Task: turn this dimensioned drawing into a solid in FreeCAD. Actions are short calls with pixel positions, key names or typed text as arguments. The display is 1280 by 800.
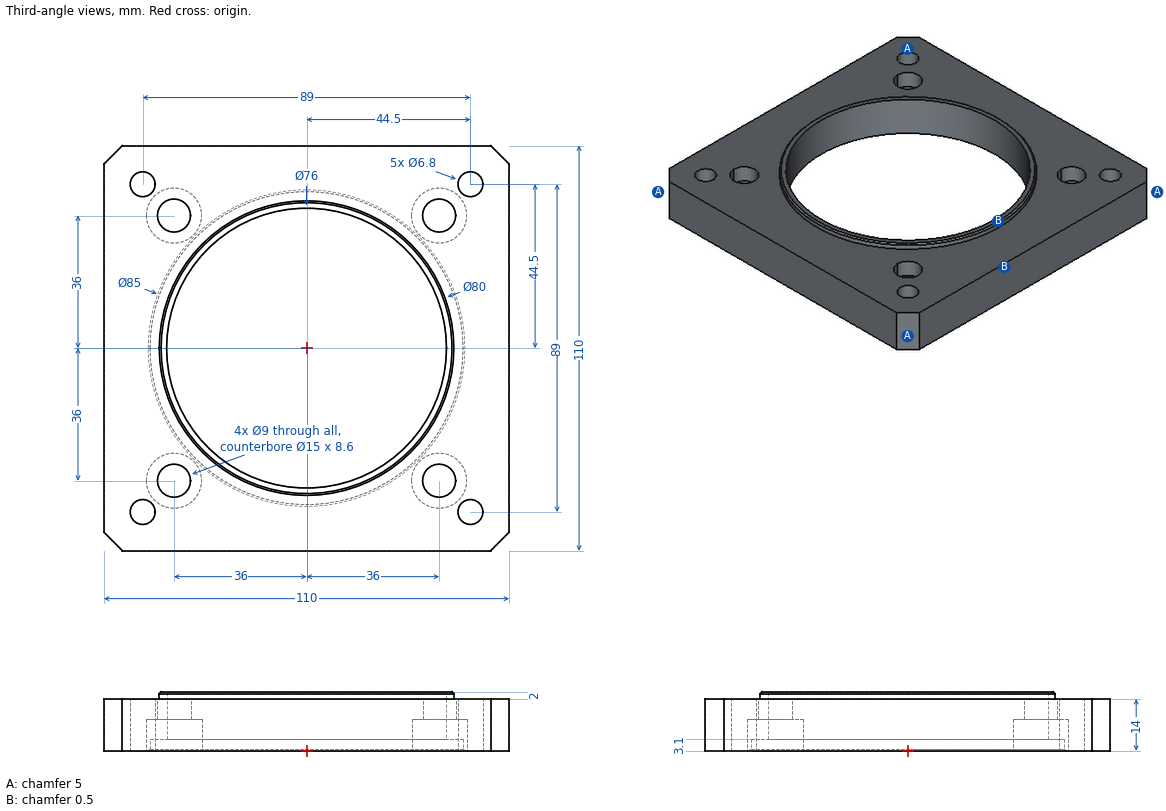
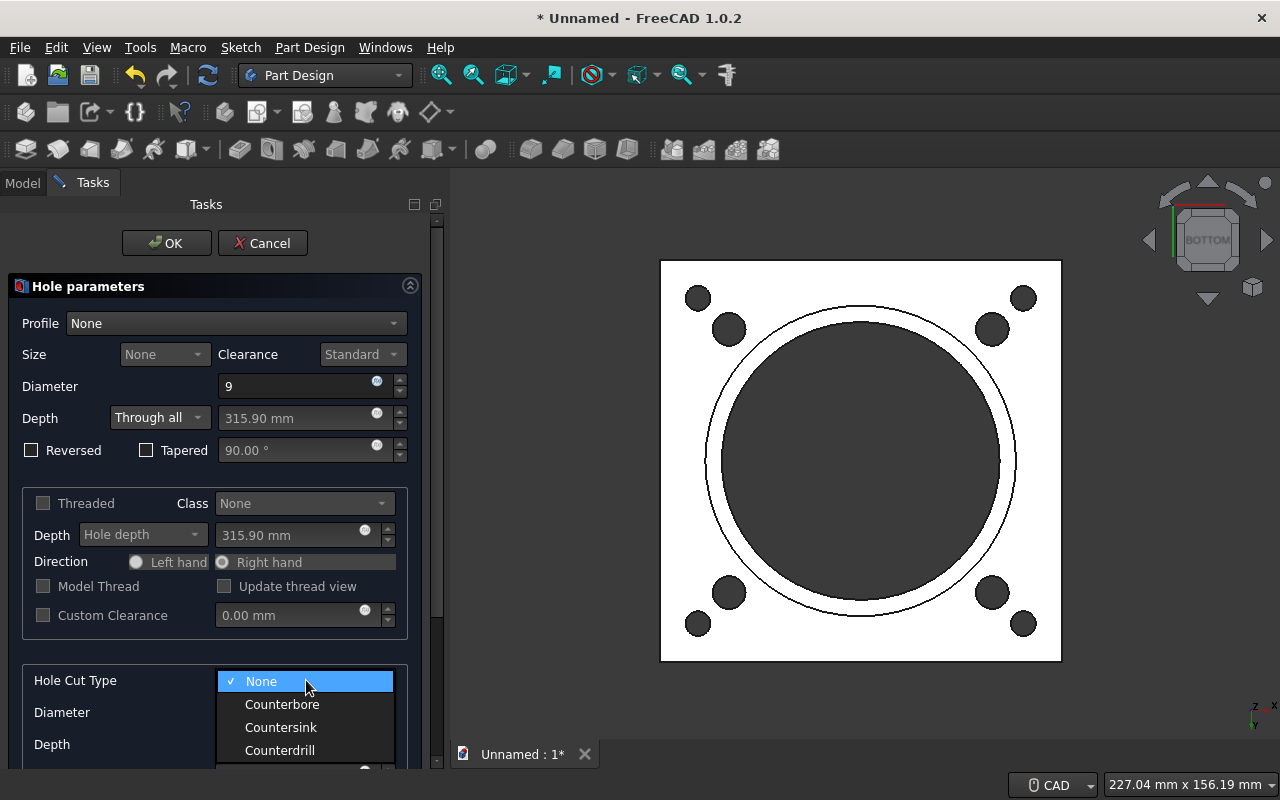
click(304, 704)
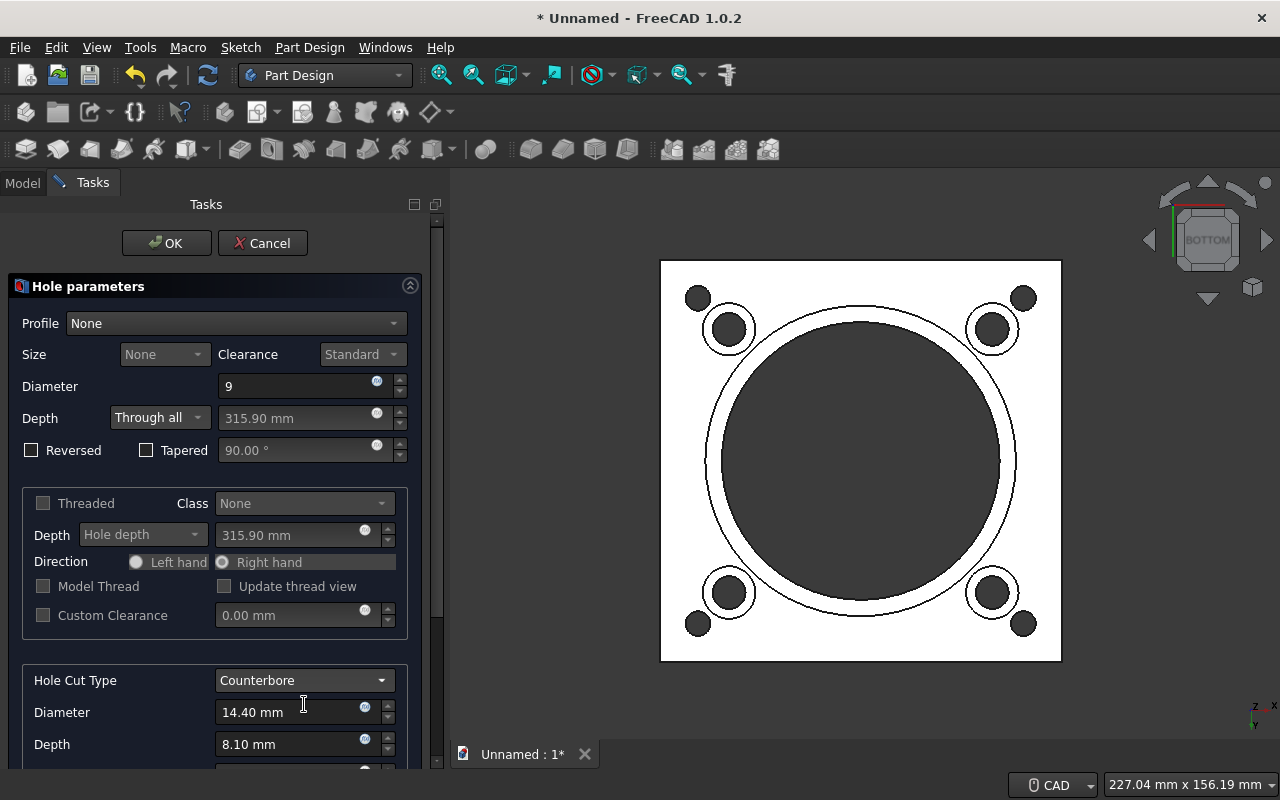
triple_click(298, 712)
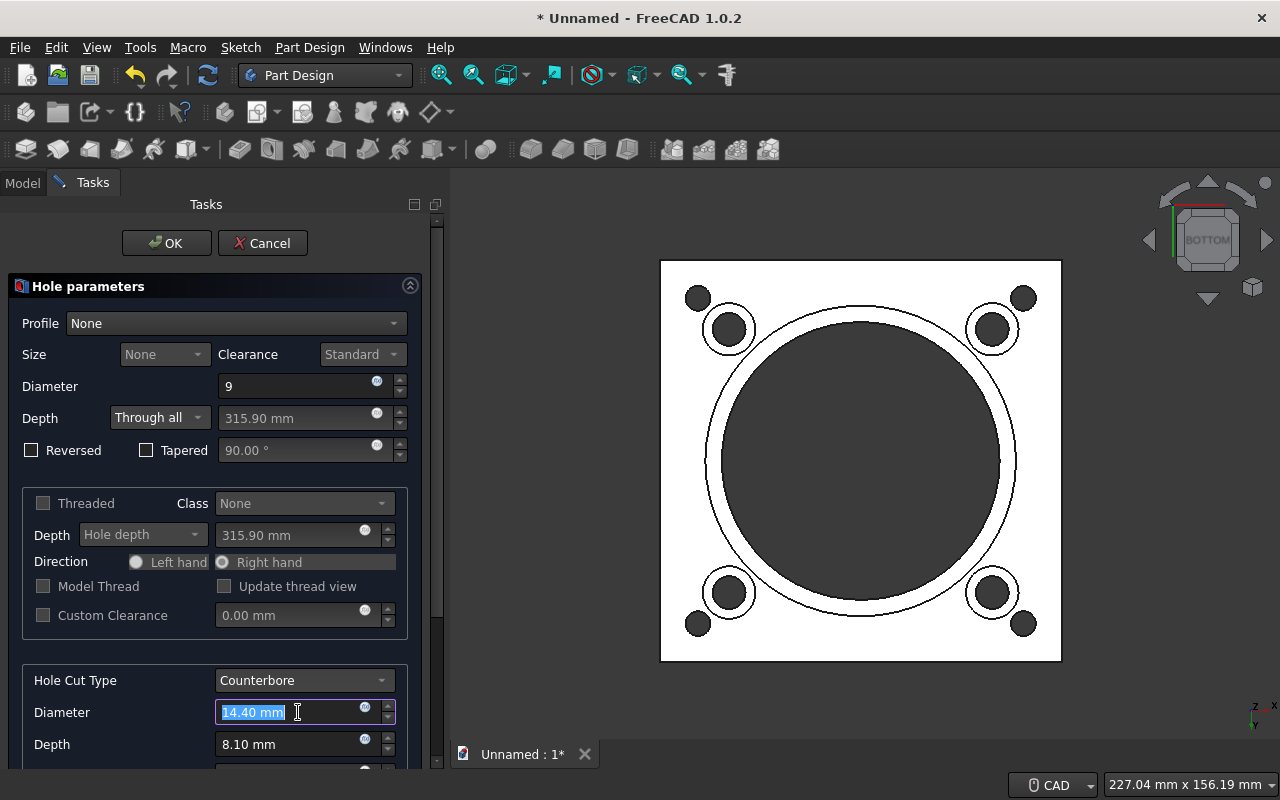
text(15)
key(Tab)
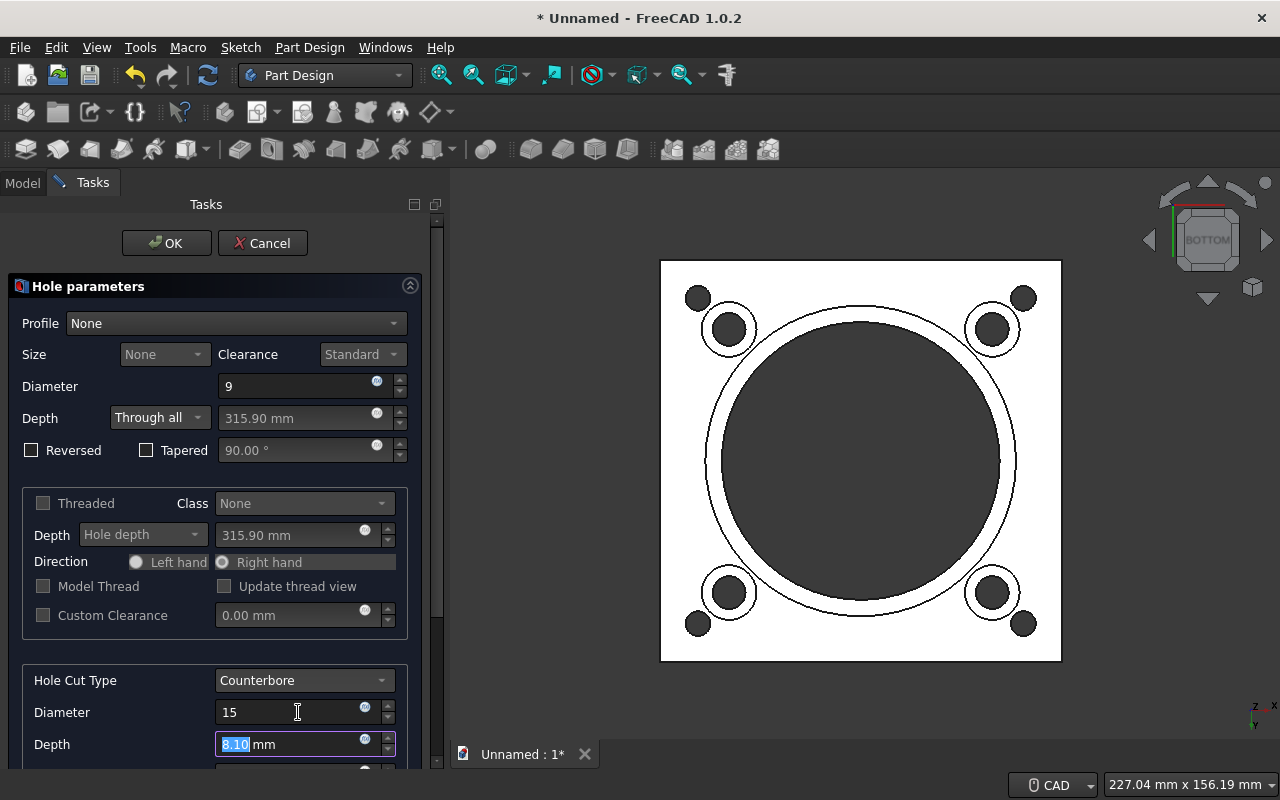
text(8.6)
key(Tab)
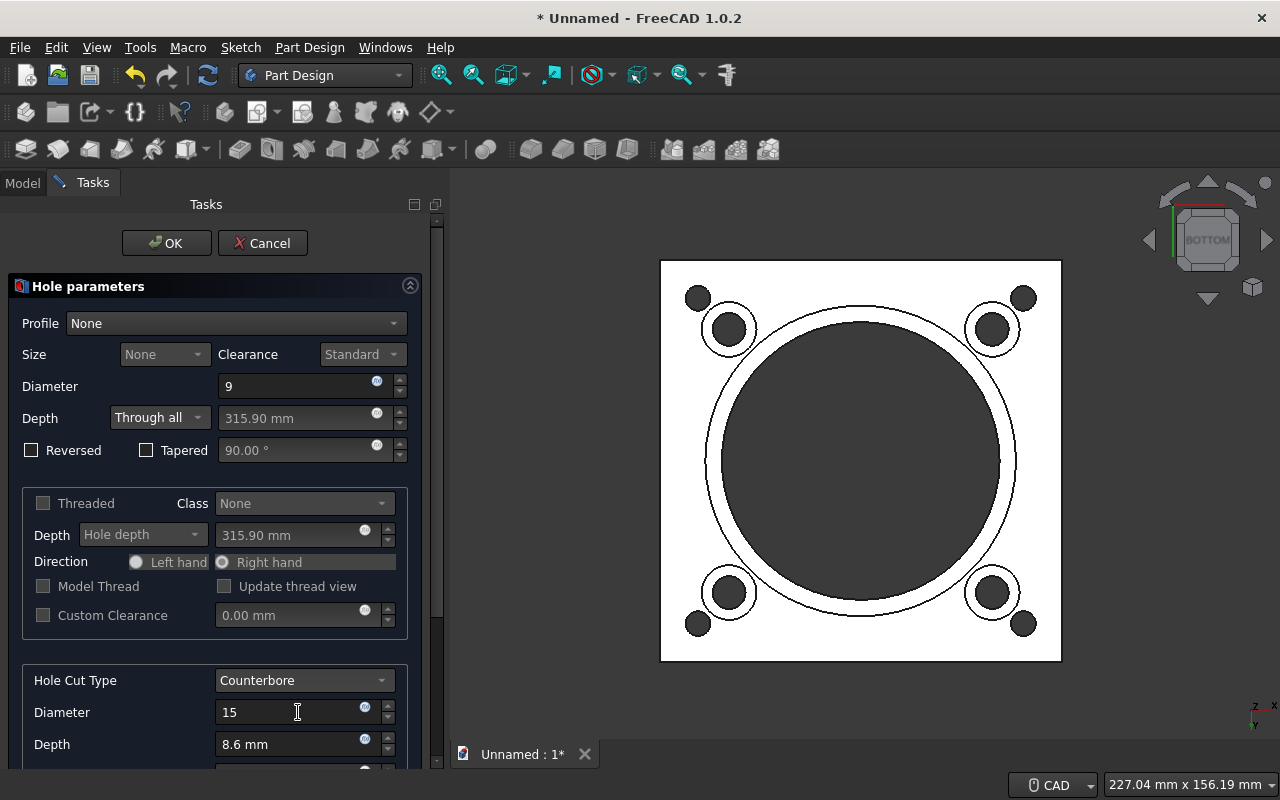
click(167, 243)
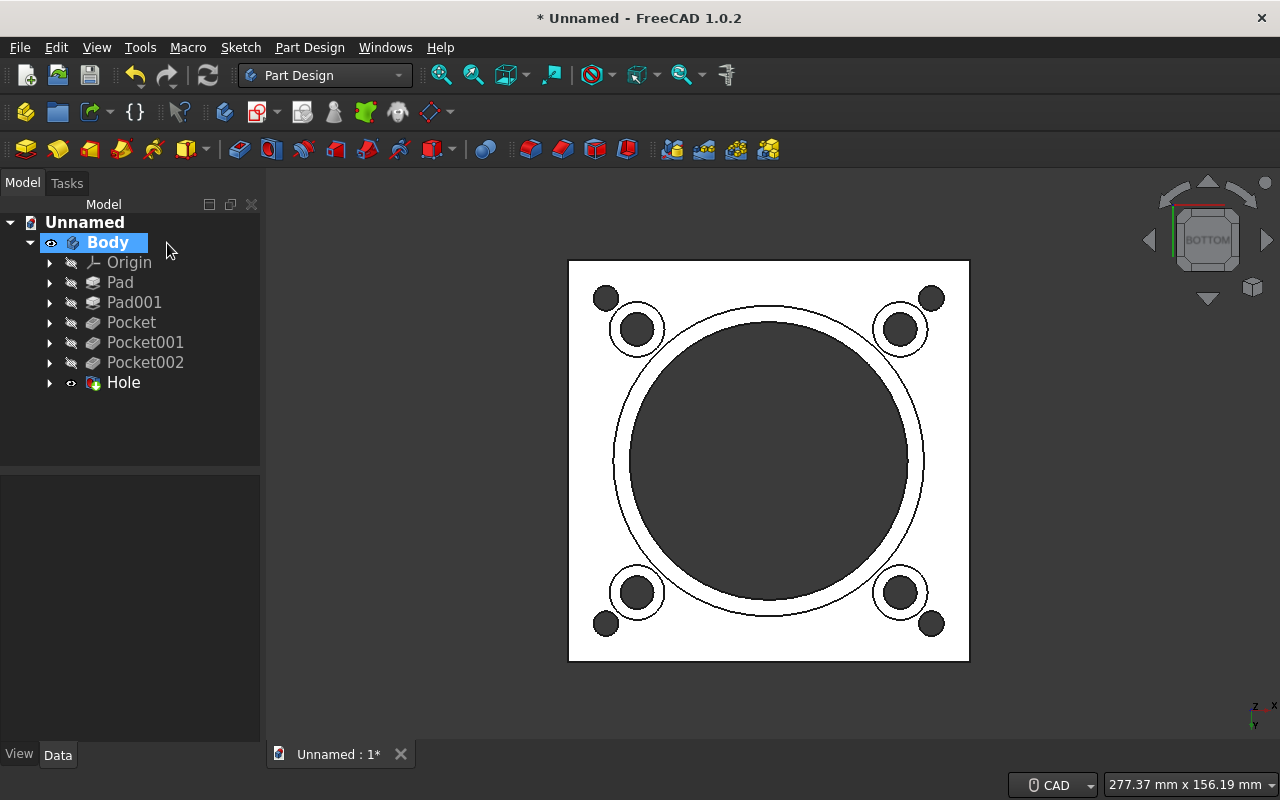
key(0)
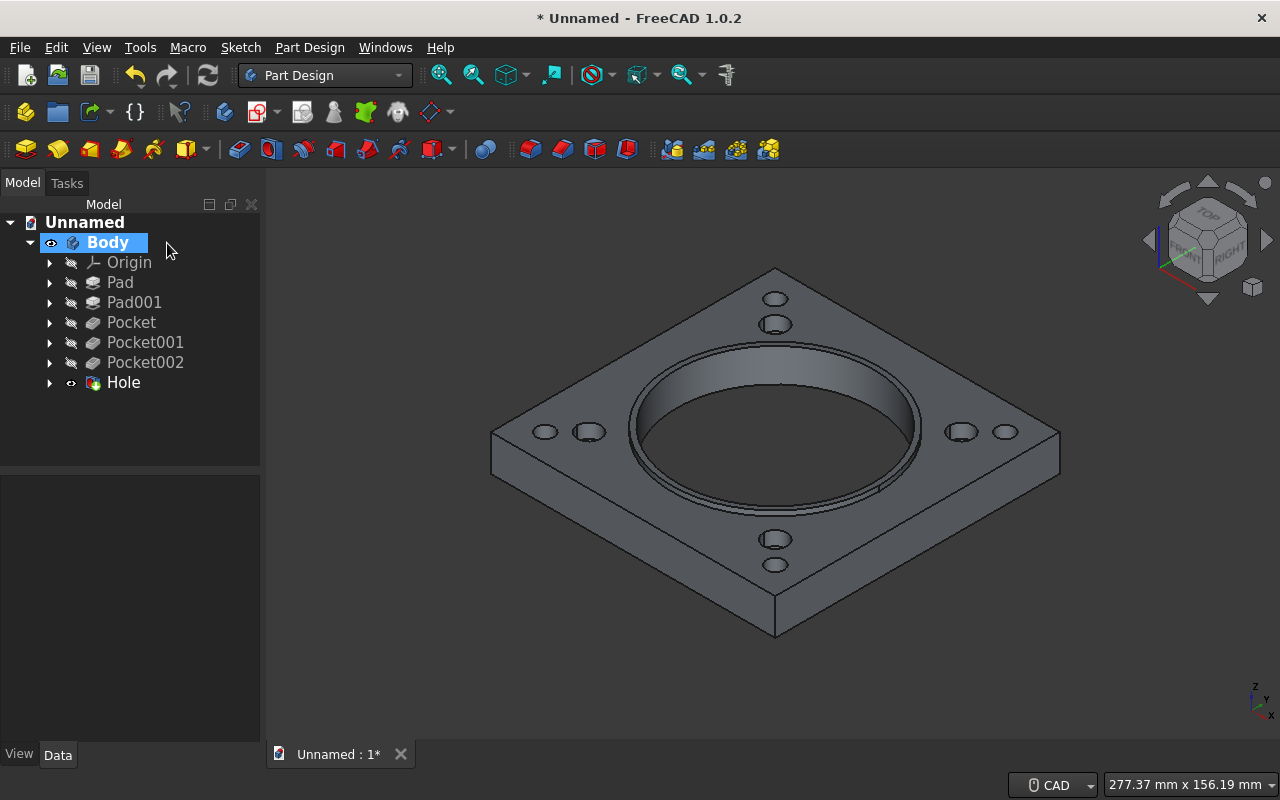
click(775, 616)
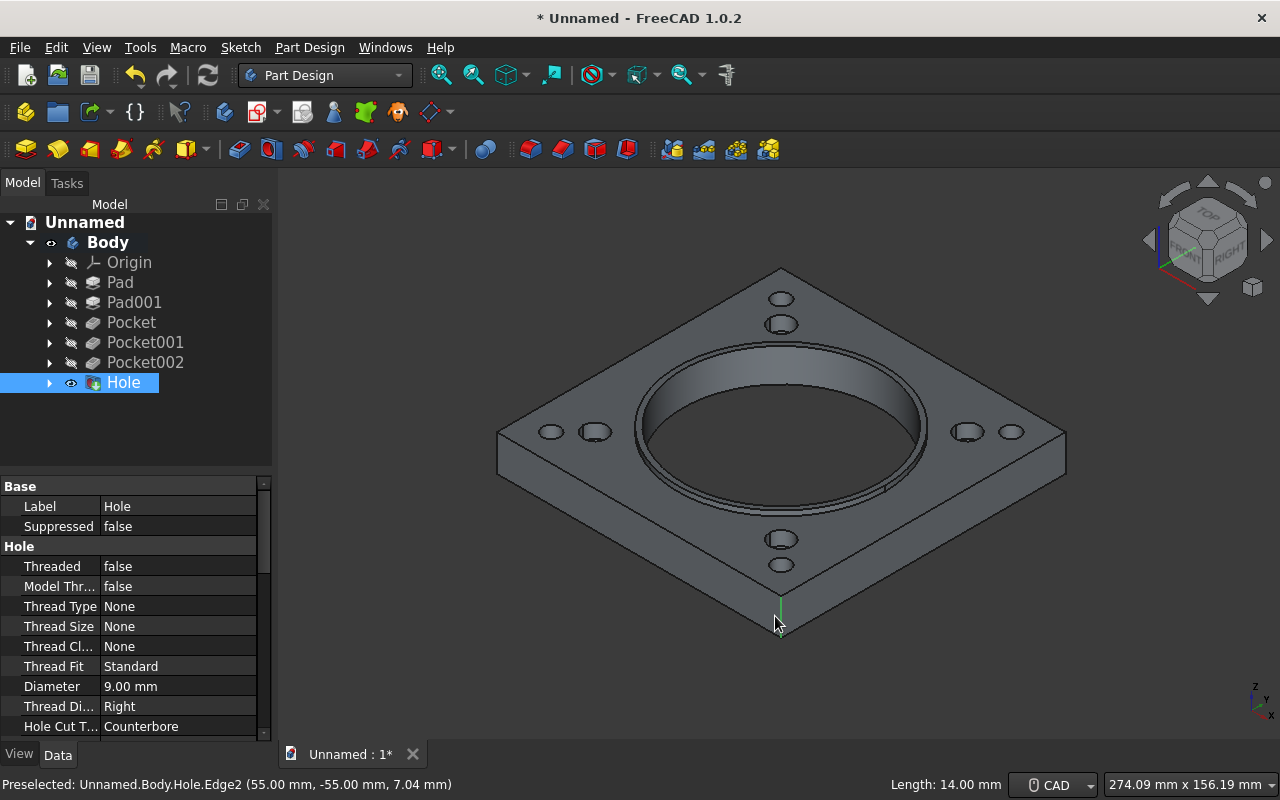
key(2)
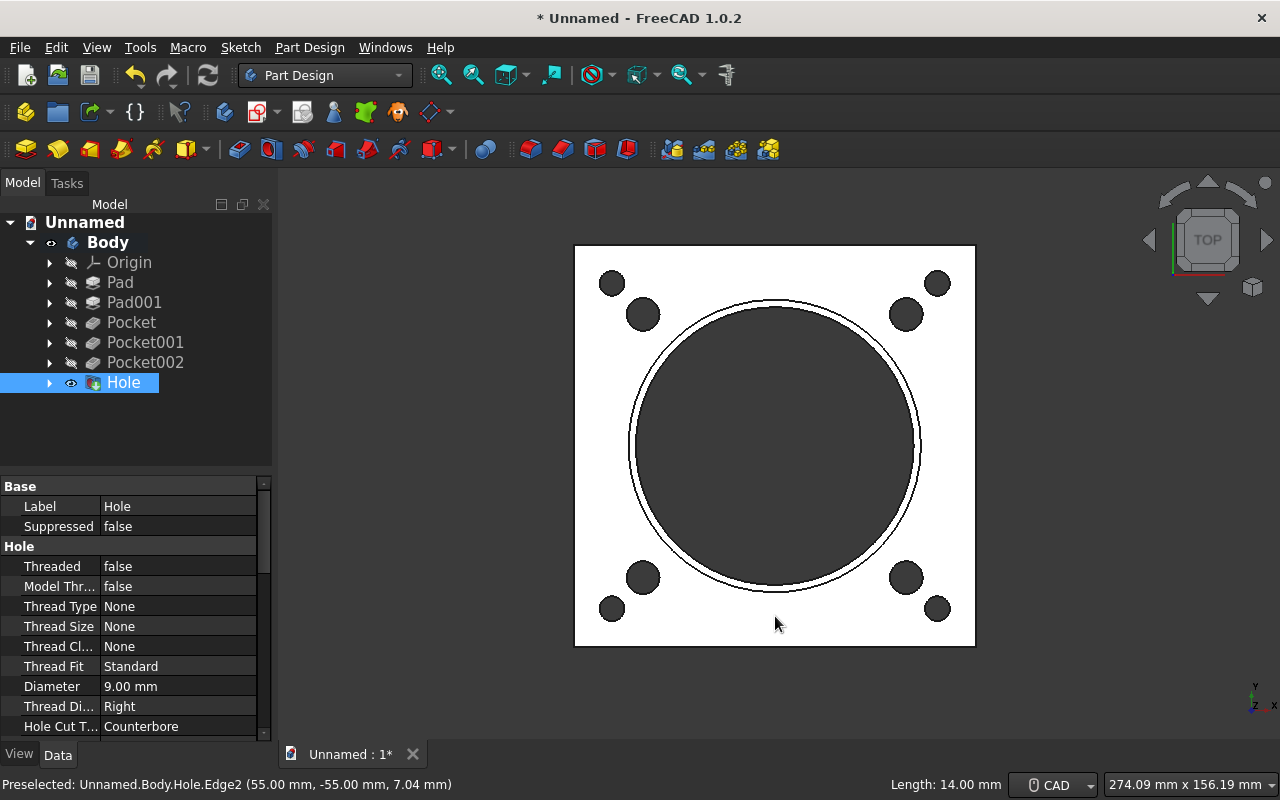
key(1)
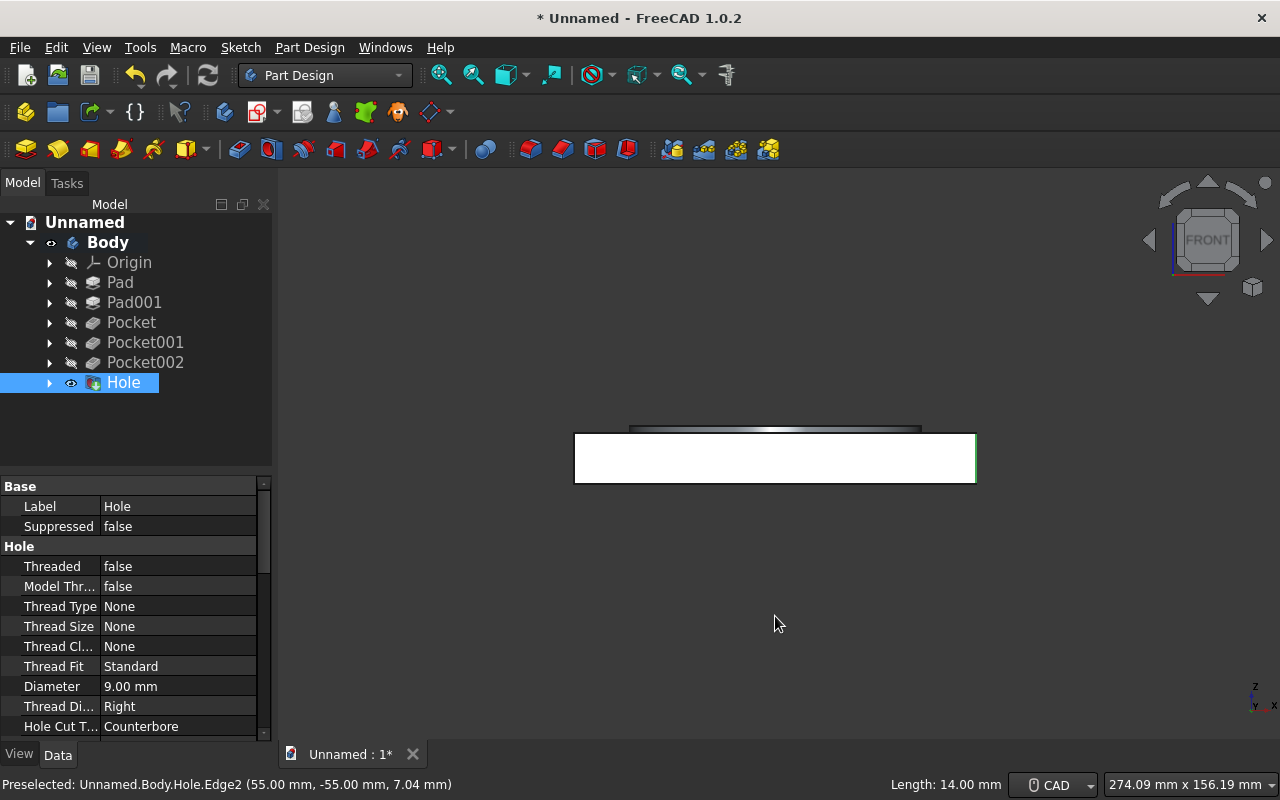
click(442, 76)